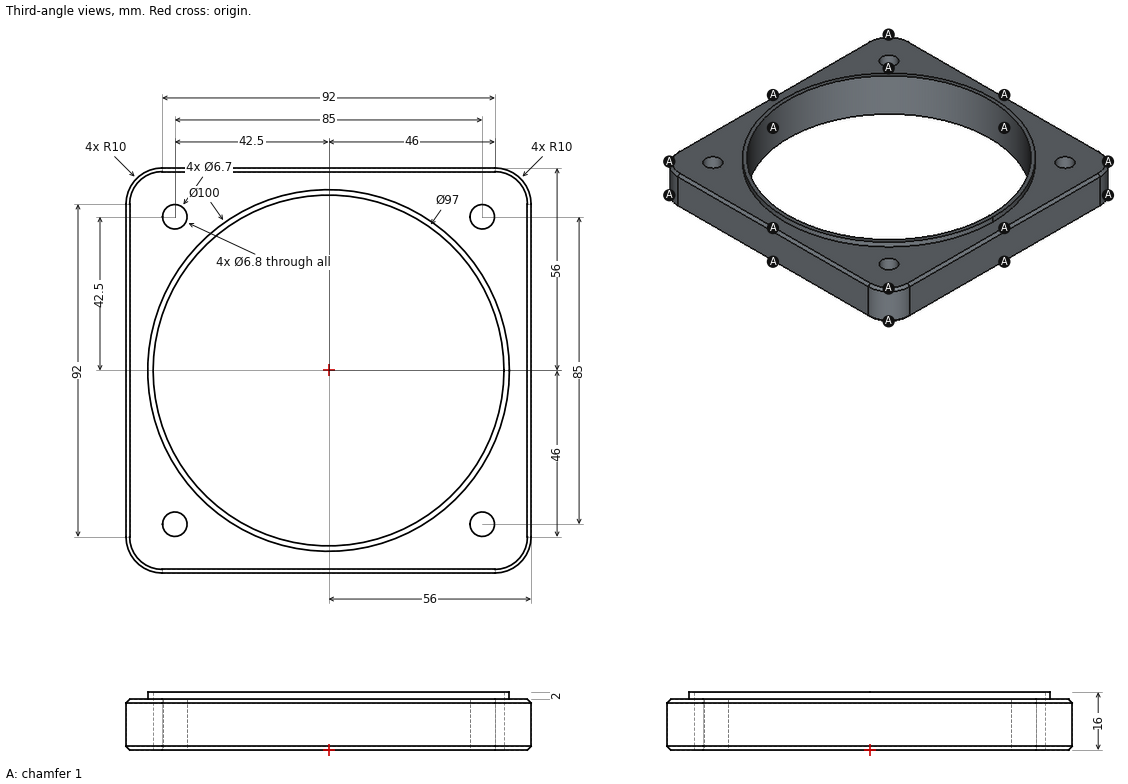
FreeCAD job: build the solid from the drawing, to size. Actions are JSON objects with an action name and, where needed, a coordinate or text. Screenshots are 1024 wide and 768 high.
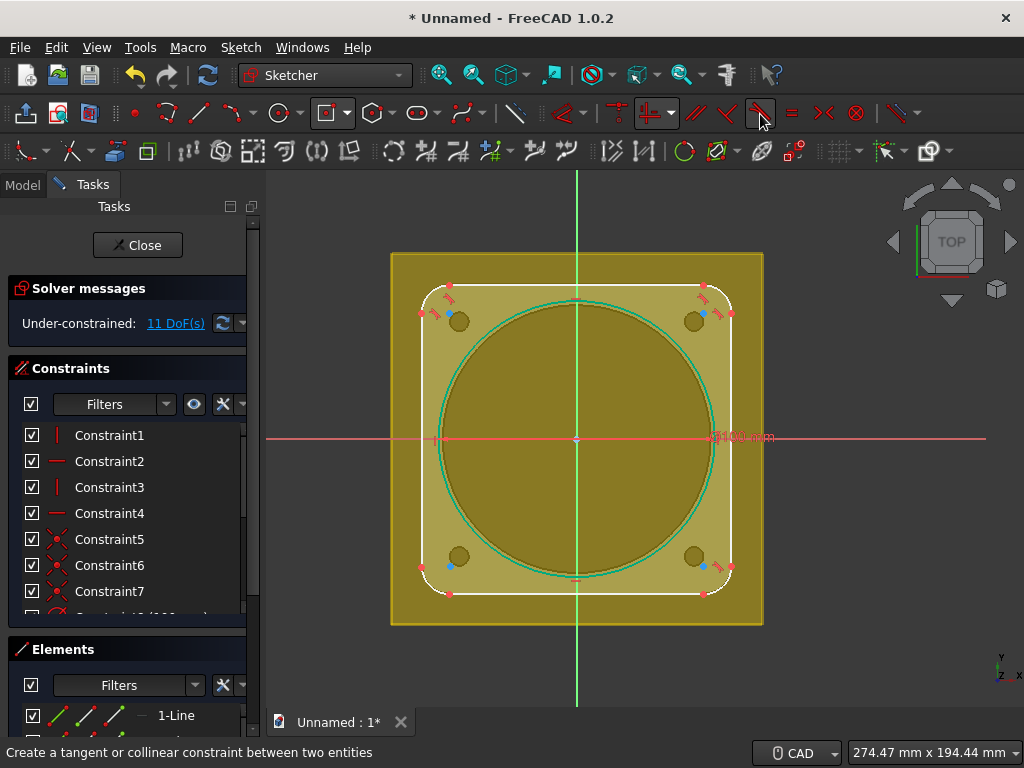
{"action": "left_click", "coordinate": [422, 389]}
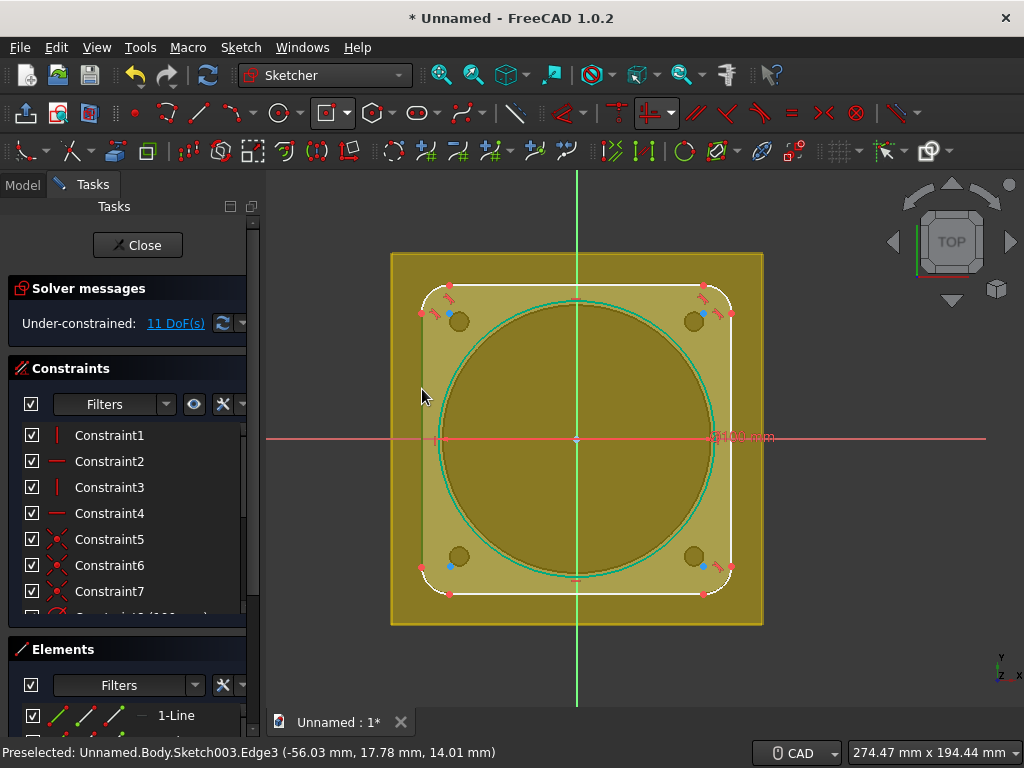
{"action": "left_click", "coordinate": [425, 580]}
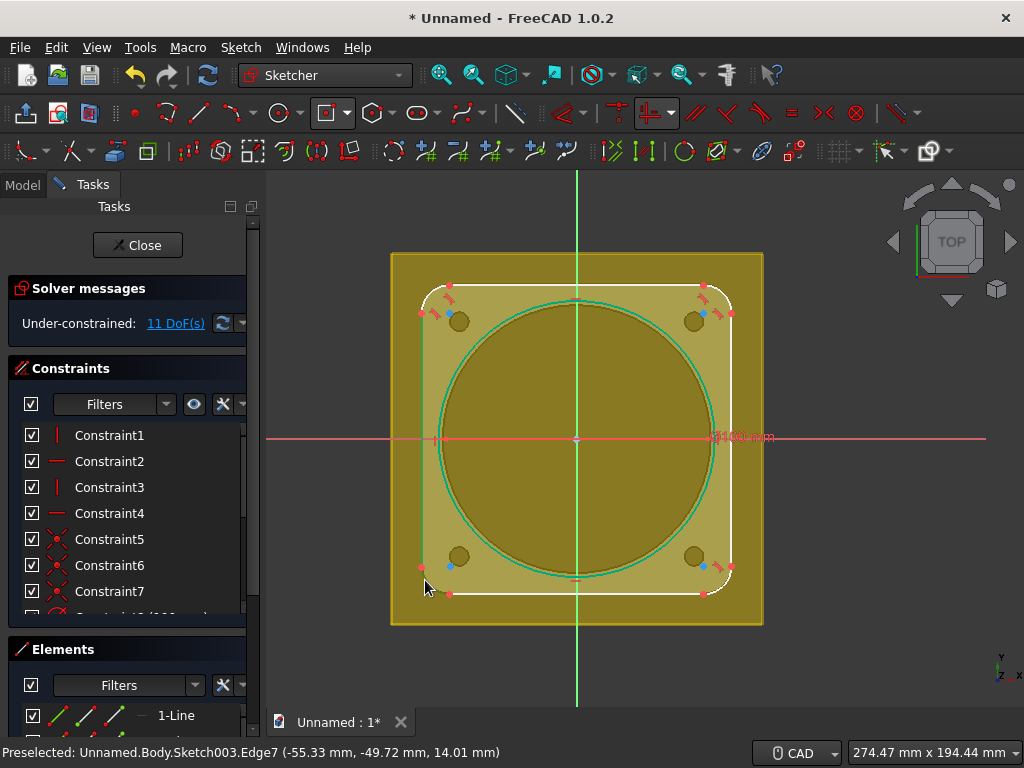
{"action": "left_click", "coordinate": [760, 114]}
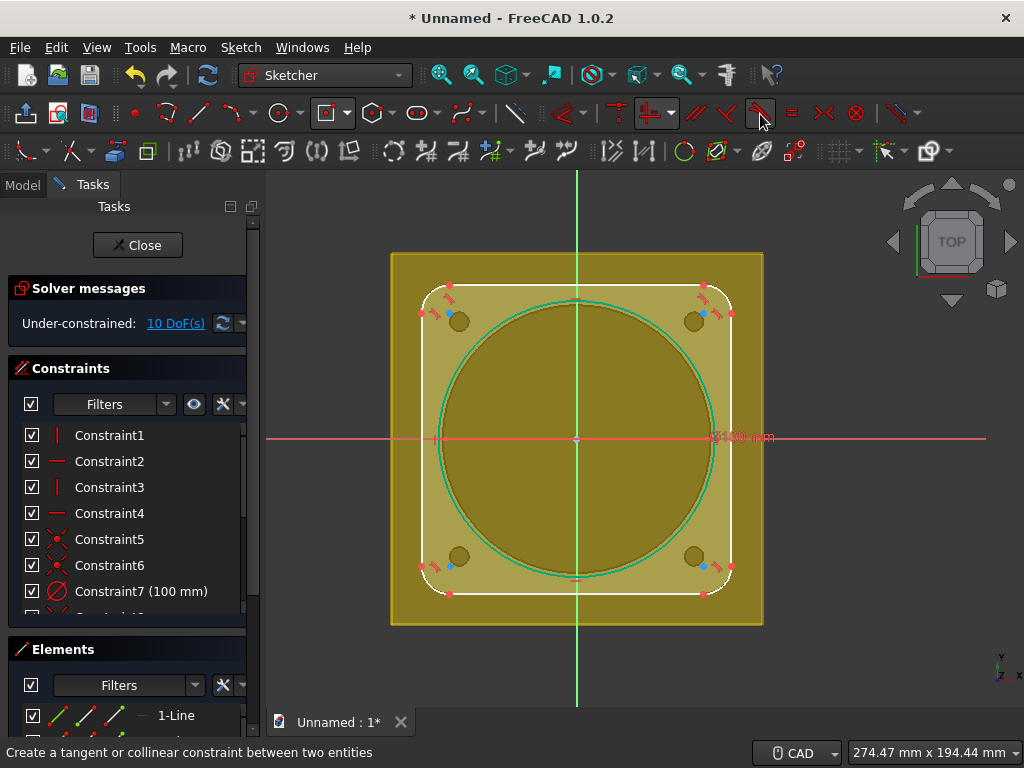
{"action": "left_click", "coordinate": [526, 594]}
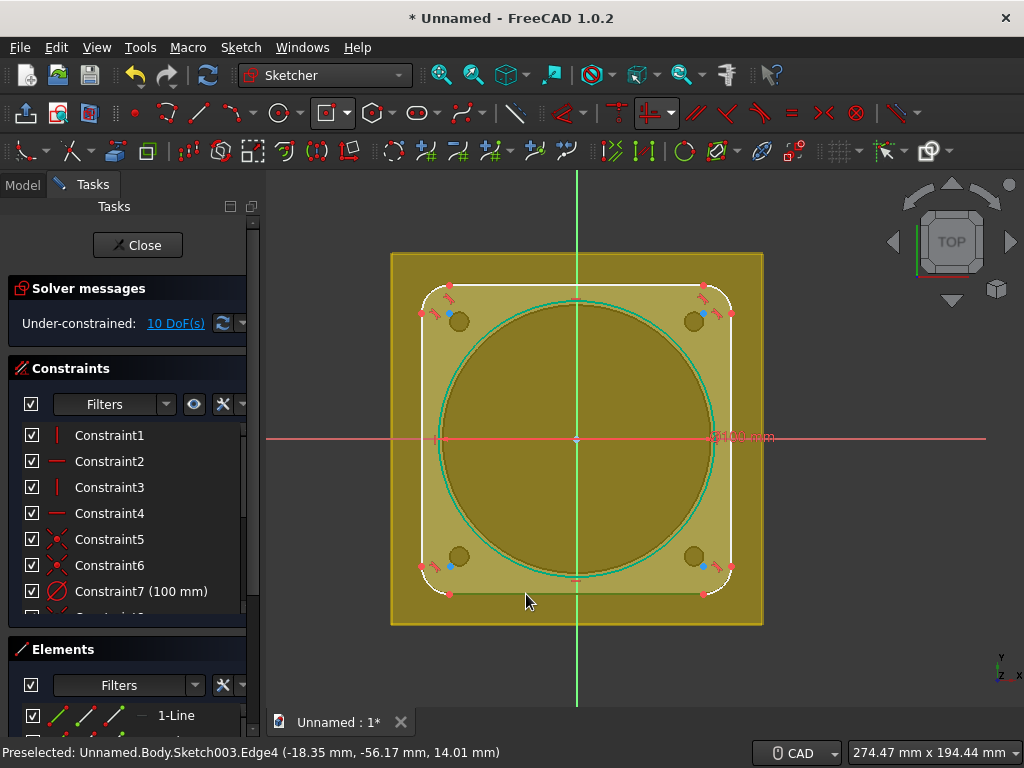
{"action": "left_click", "coordinate": [425, 579]}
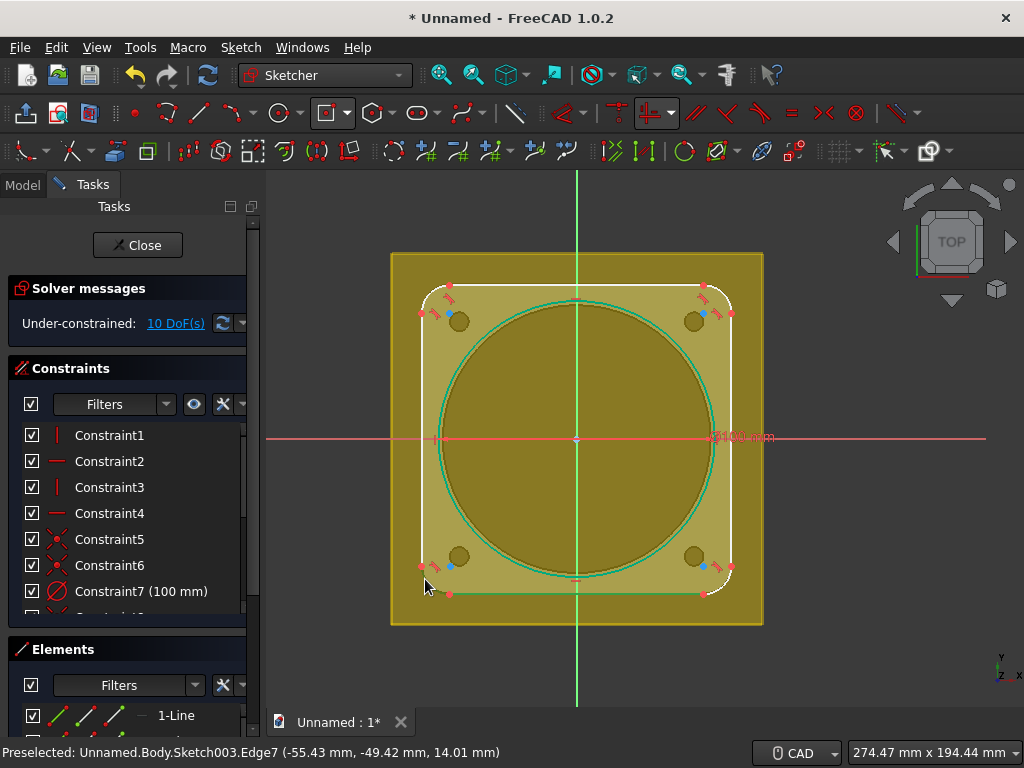
{"action": "left_click", "coordinate": [760, 114]}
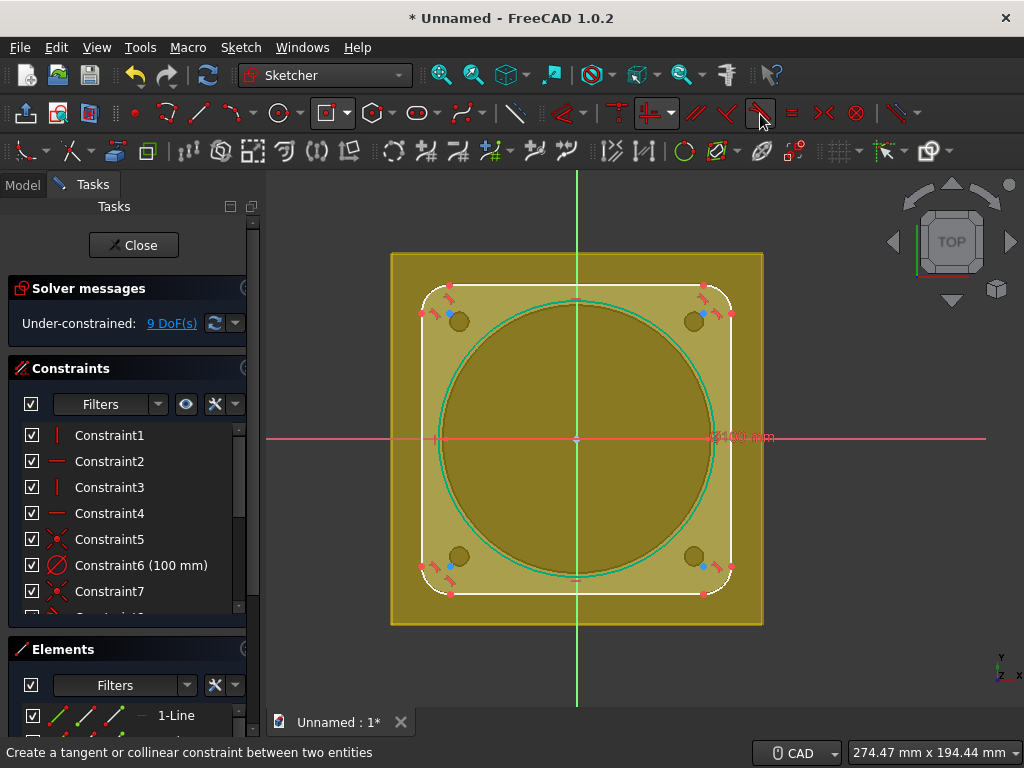
{"action": "left_click", "coordinate": [526, 594]}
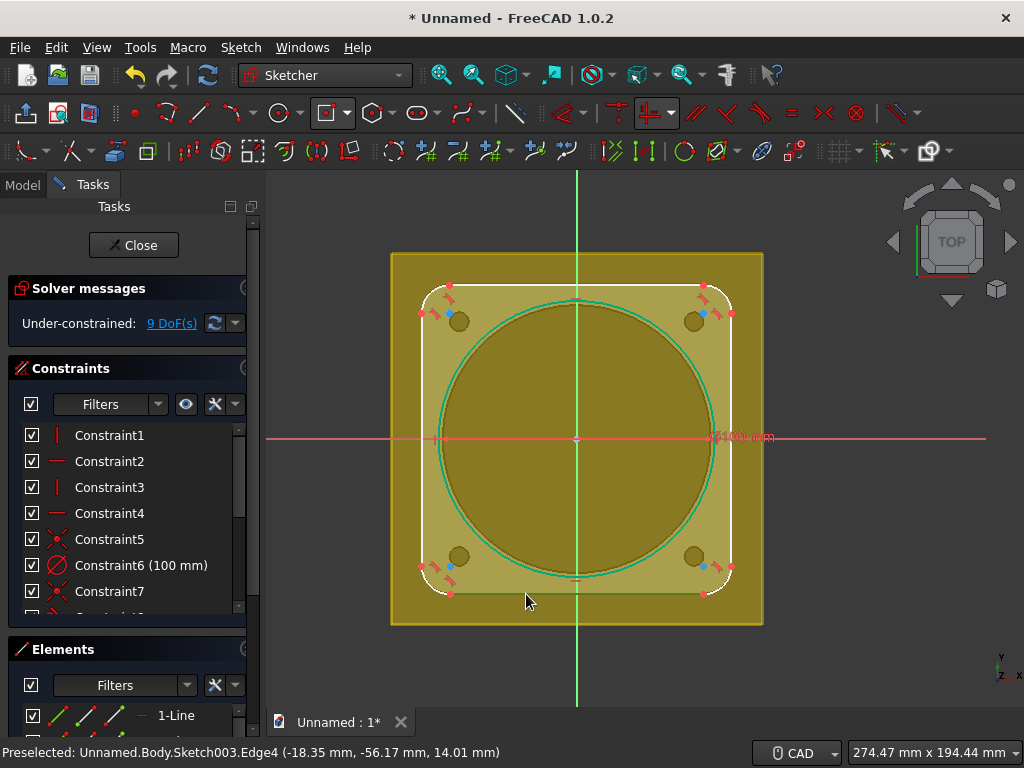
{"action": "left_click", "coordinate": [716, 591]}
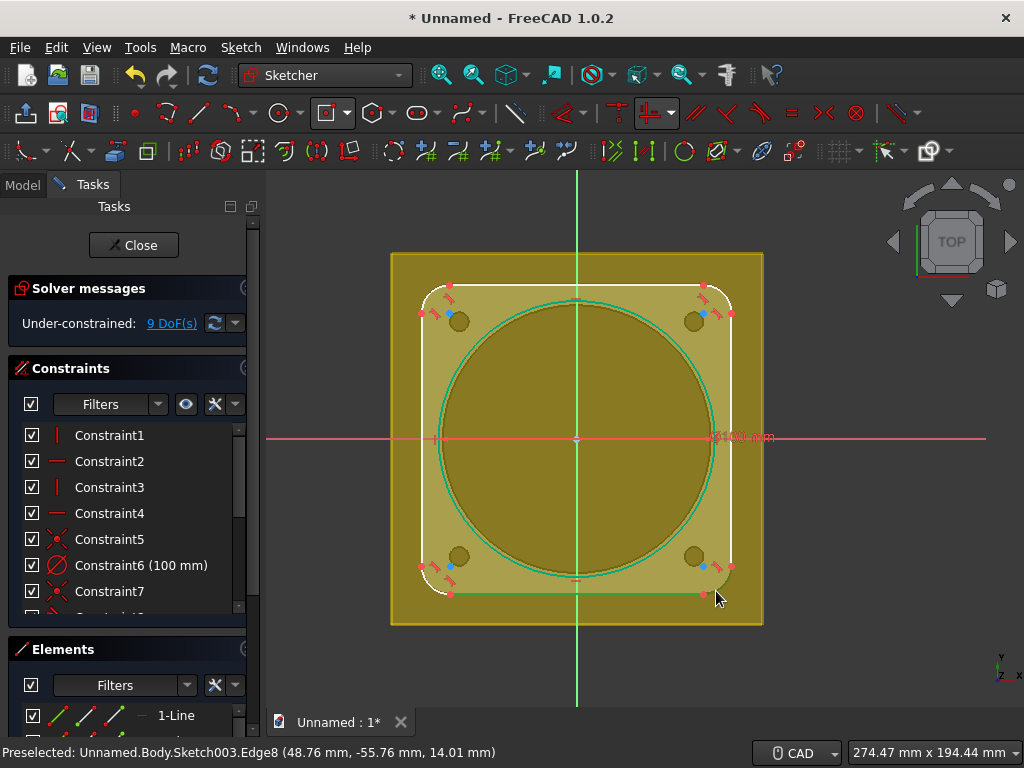
{"action": "left_click", "coordinate": [760, 114]}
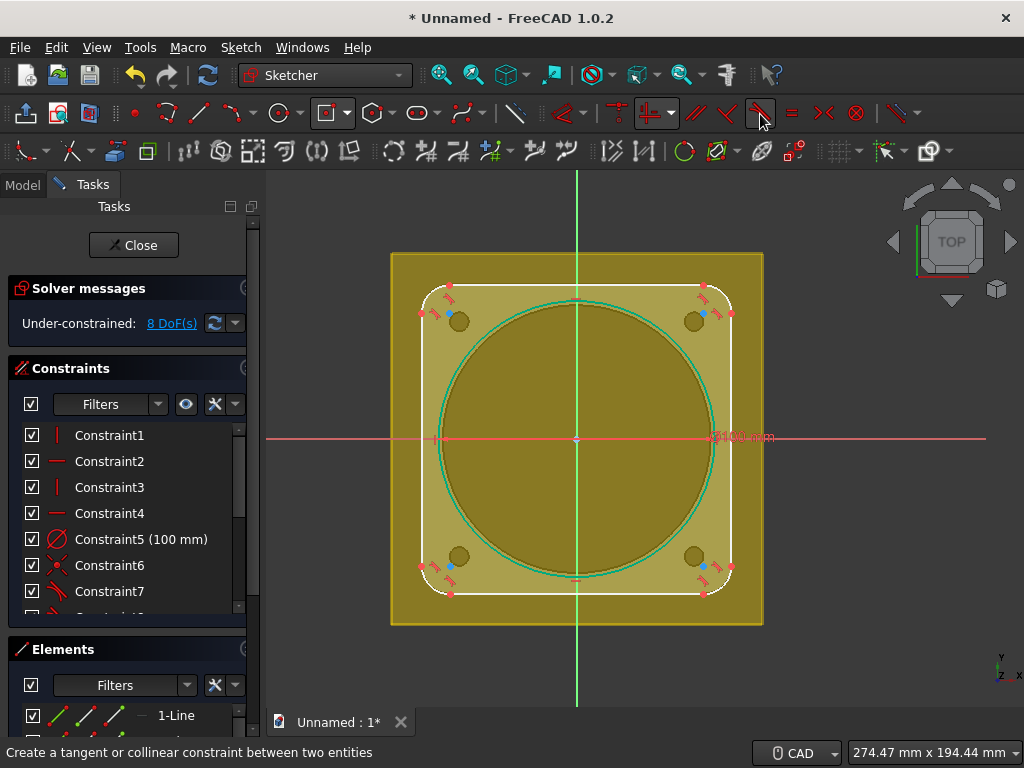
{"action": "left_click", "coordinate": [728, 301]}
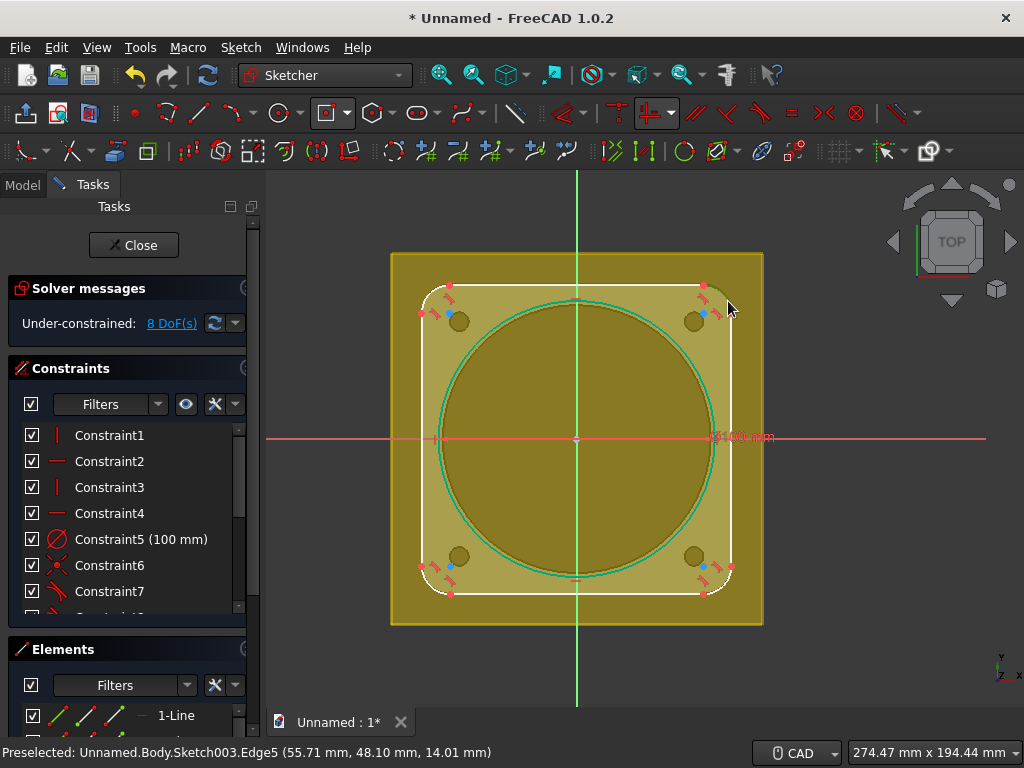
{"action": "left_click", "coordinate": [437, 288]}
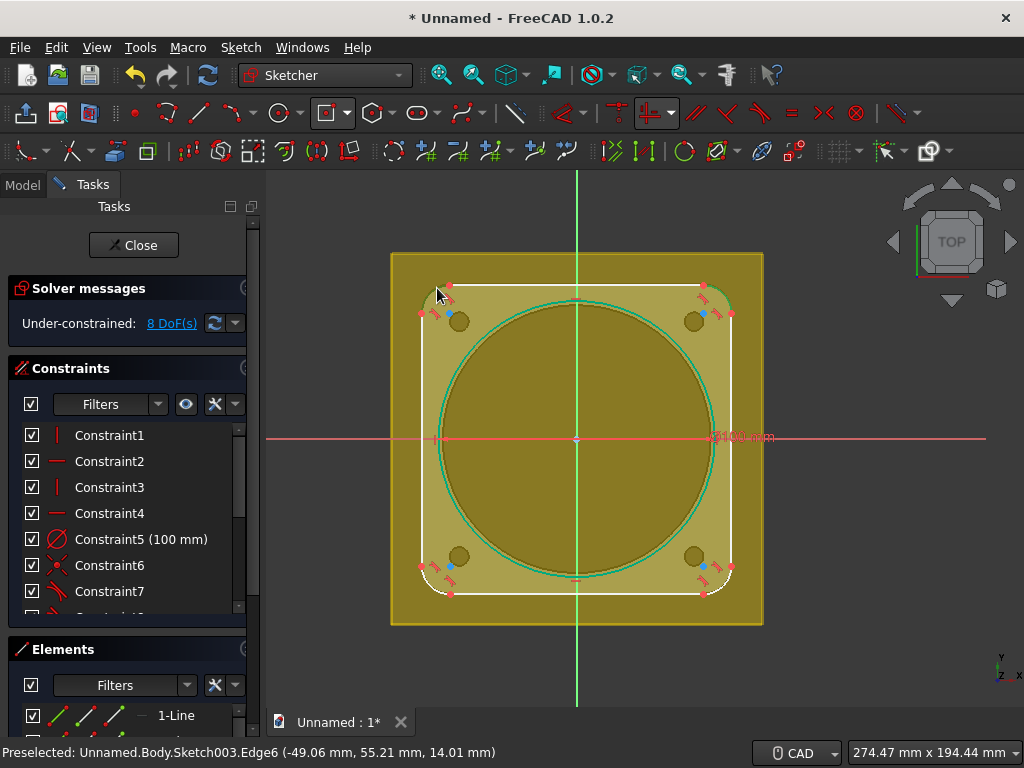
{"action": "left_click", "coordinate": [425, 579]}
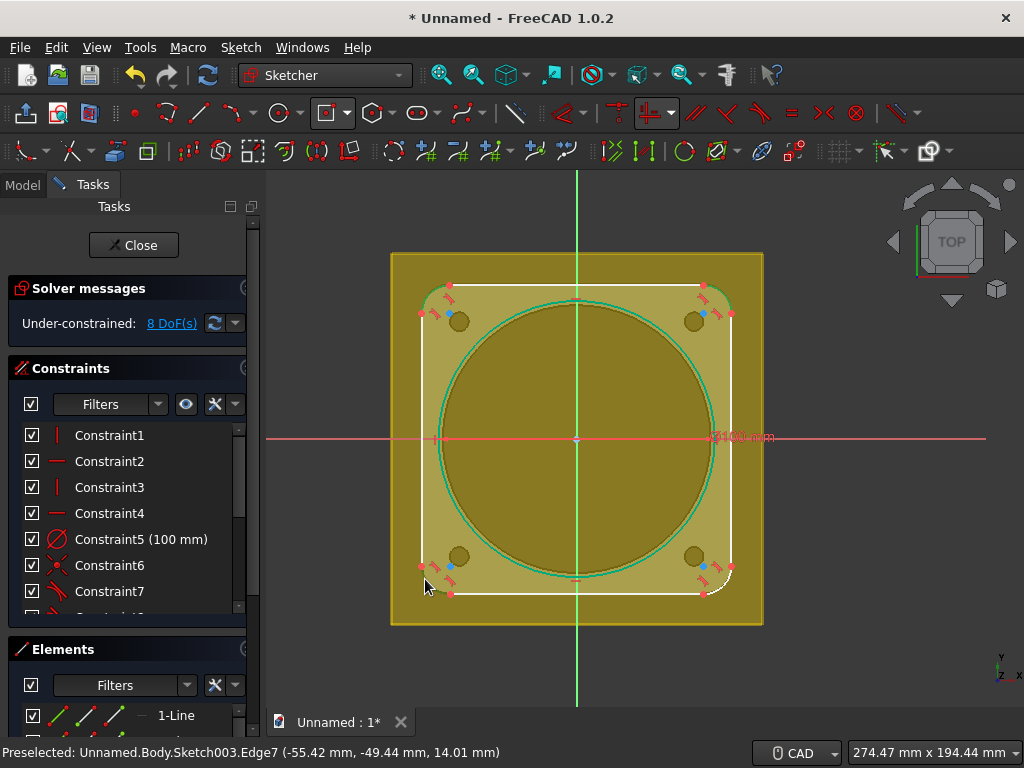
{"action": "left_click", "coordinate": [716, 591]}